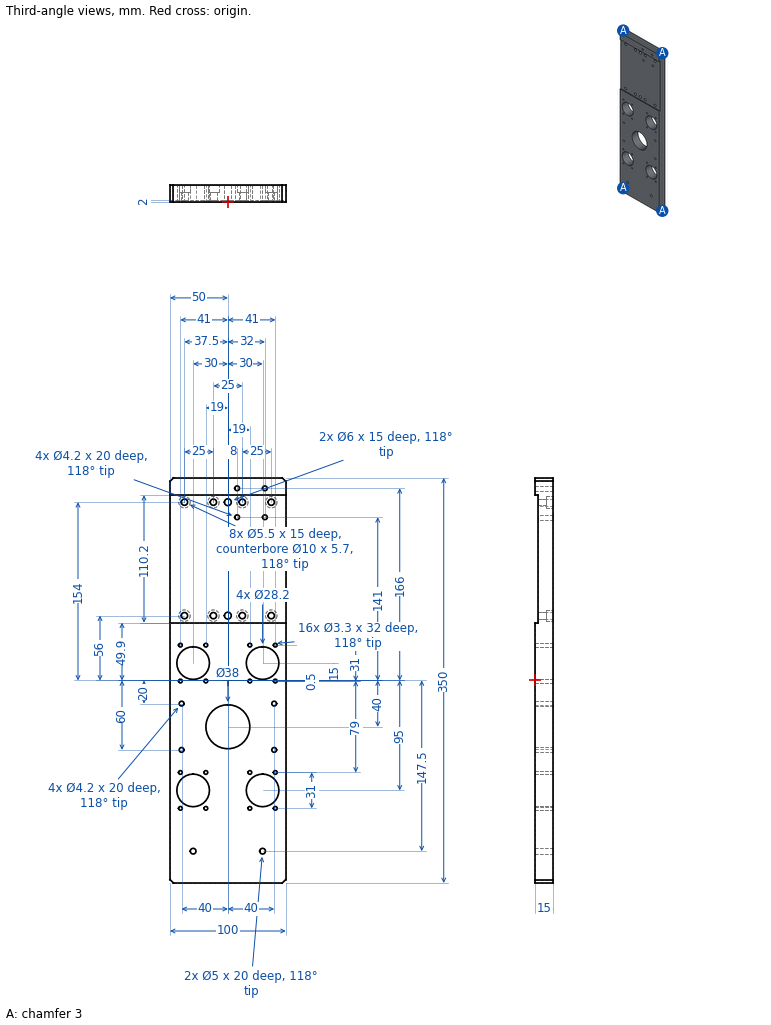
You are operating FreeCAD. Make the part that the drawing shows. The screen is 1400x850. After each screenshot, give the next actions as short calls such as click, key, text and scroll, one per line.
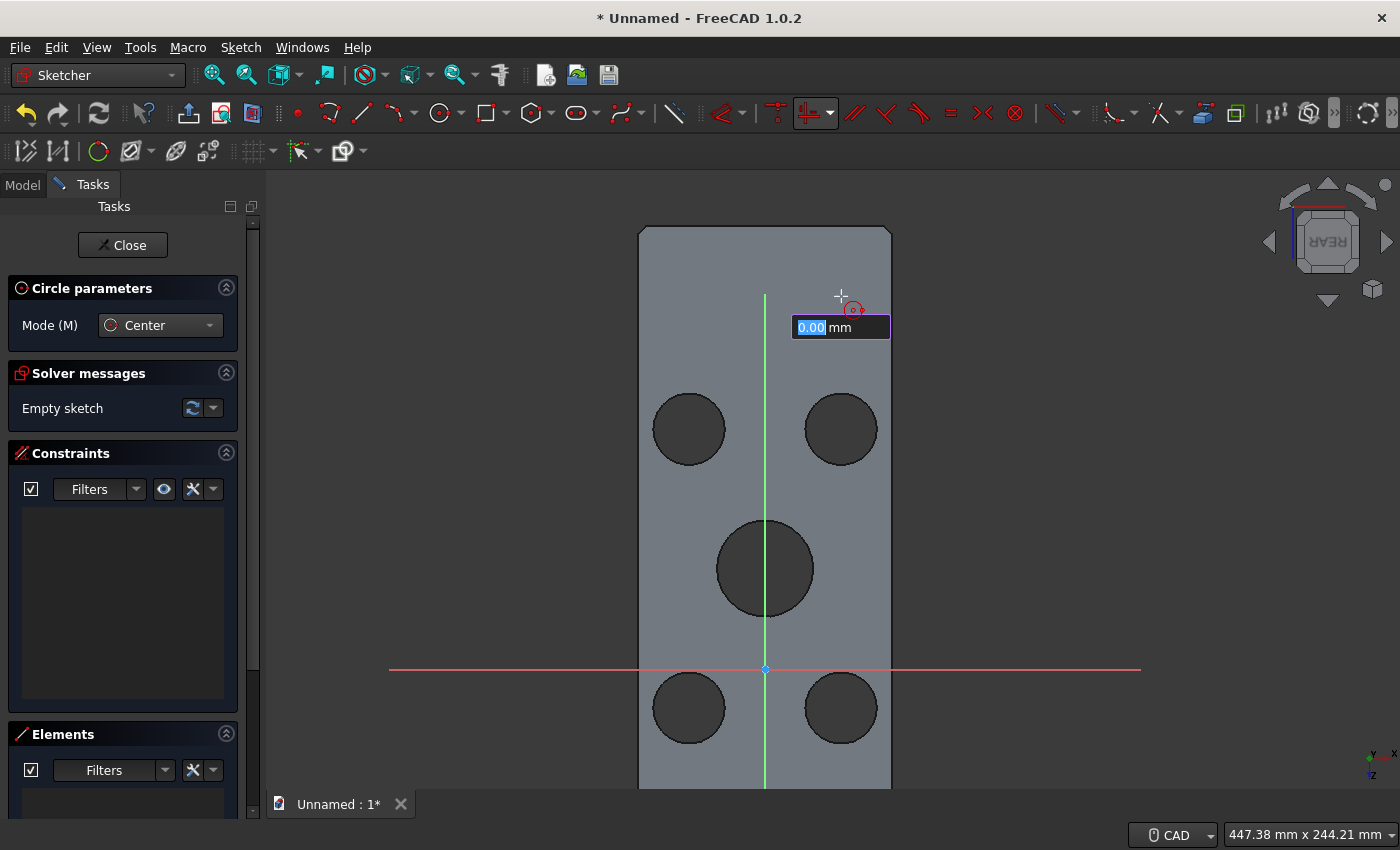
scroll(846, 292, up, 5)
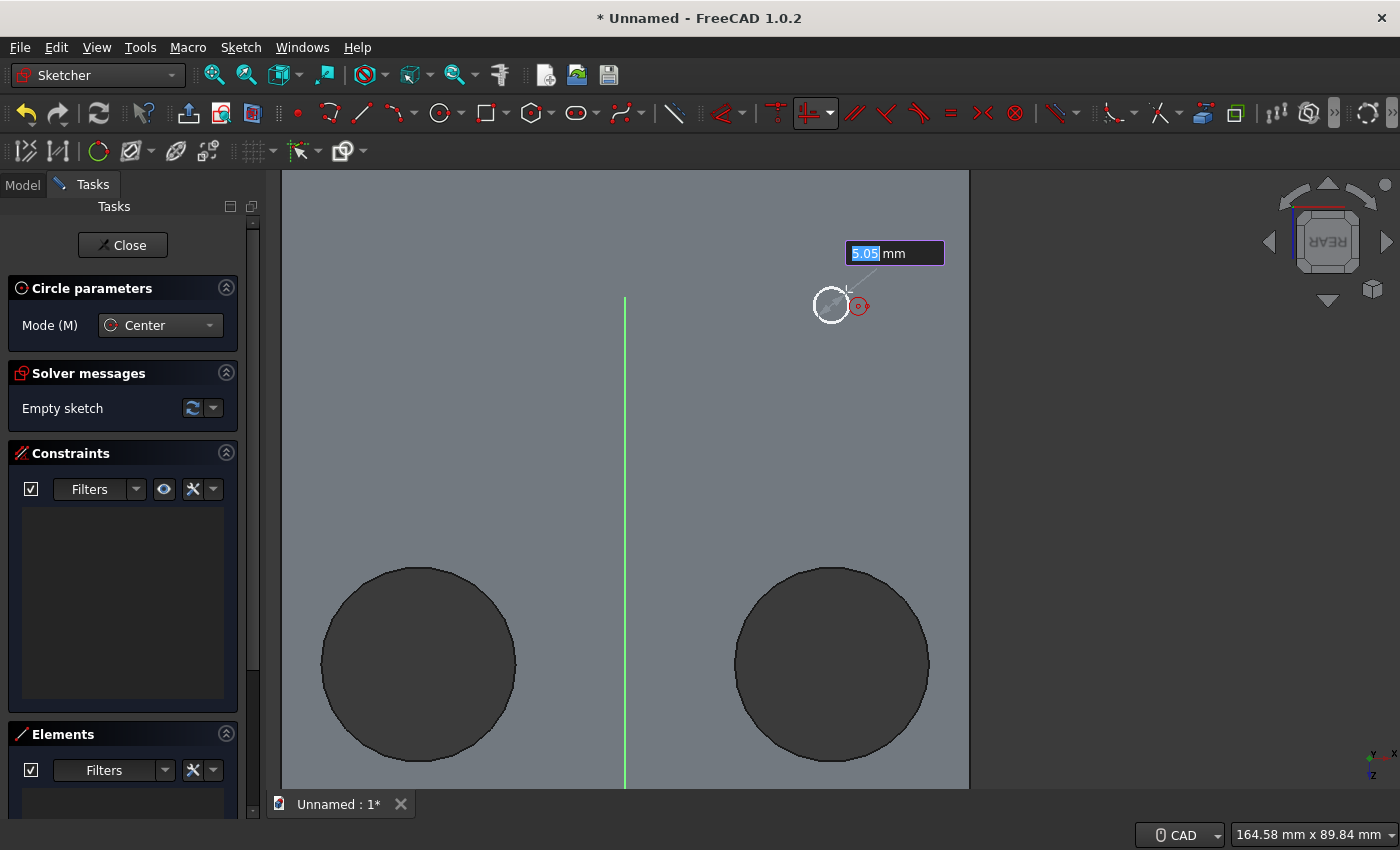
click(844, 291)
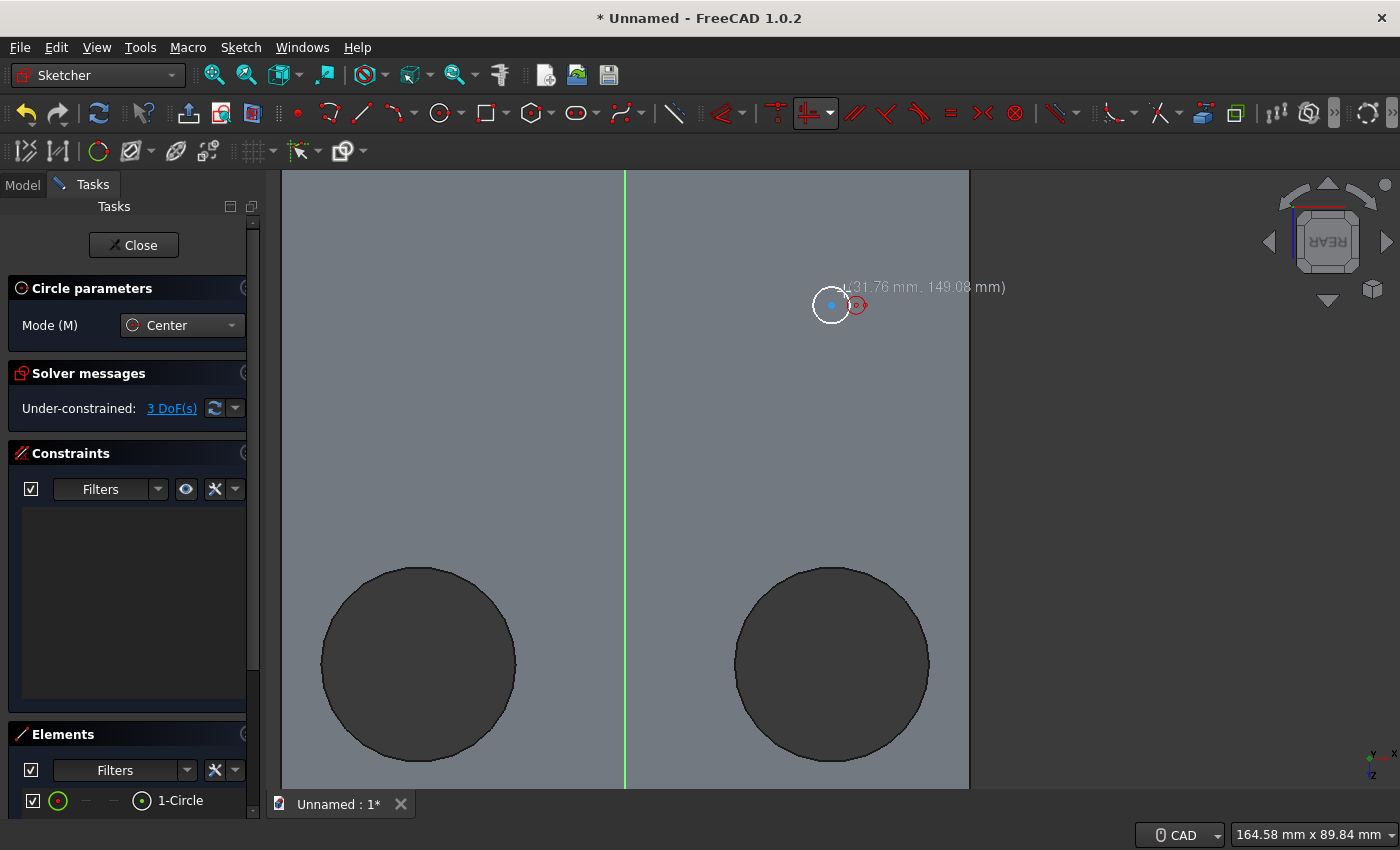
scroll(418, 303, up, 2)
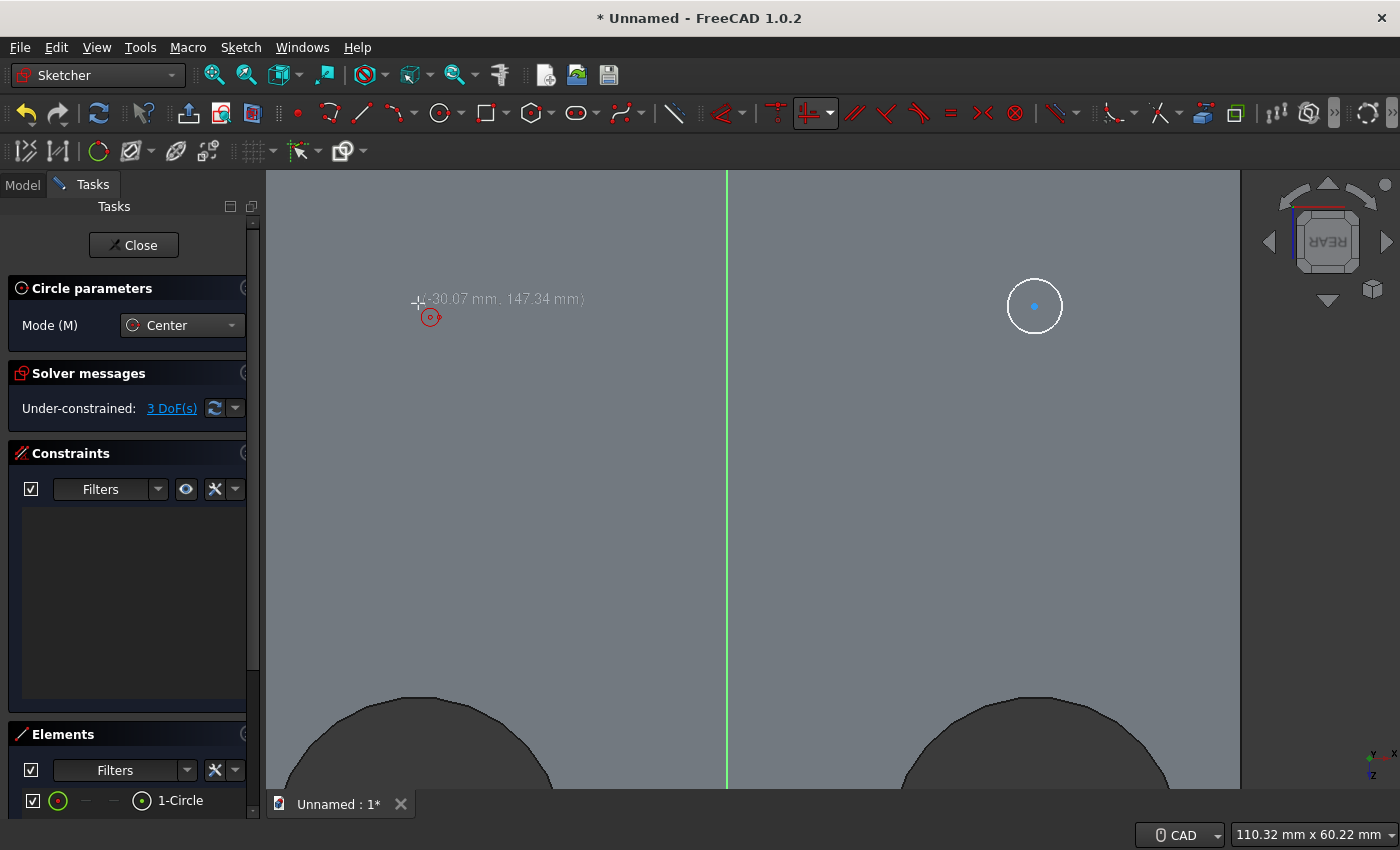
scroll(777, 293, down, 7)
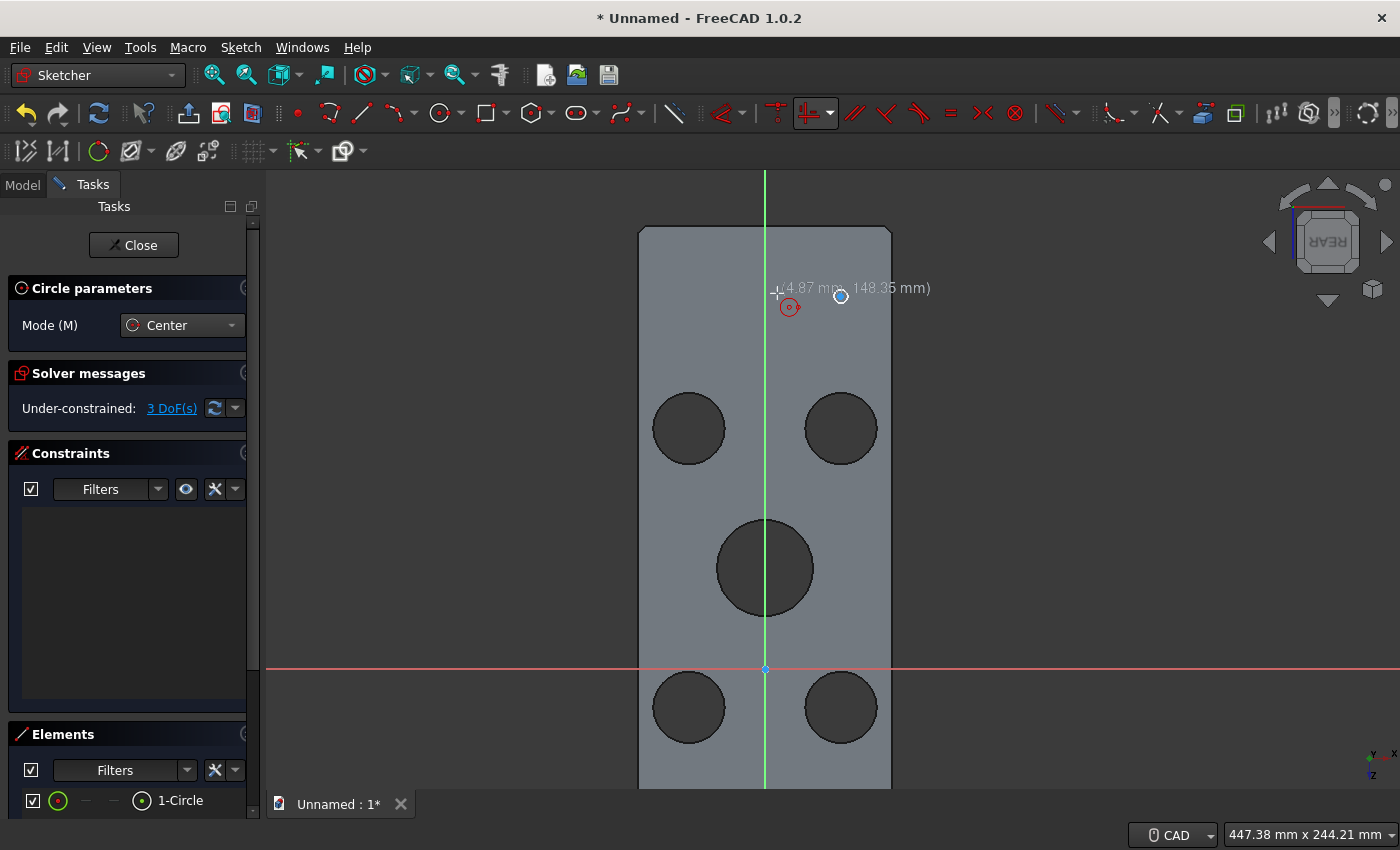
click(689, 296)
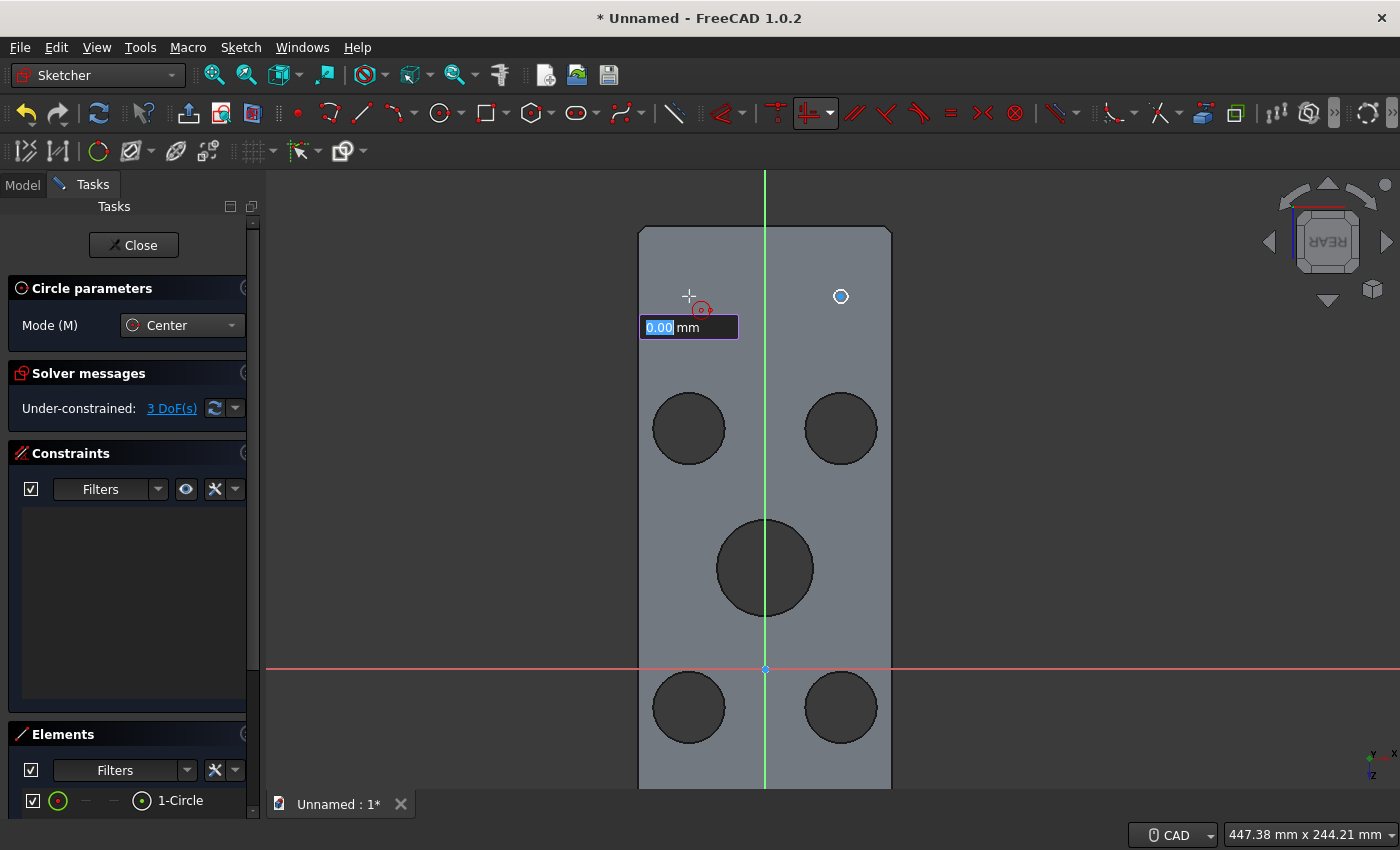
scroll(693, 291, up, 5)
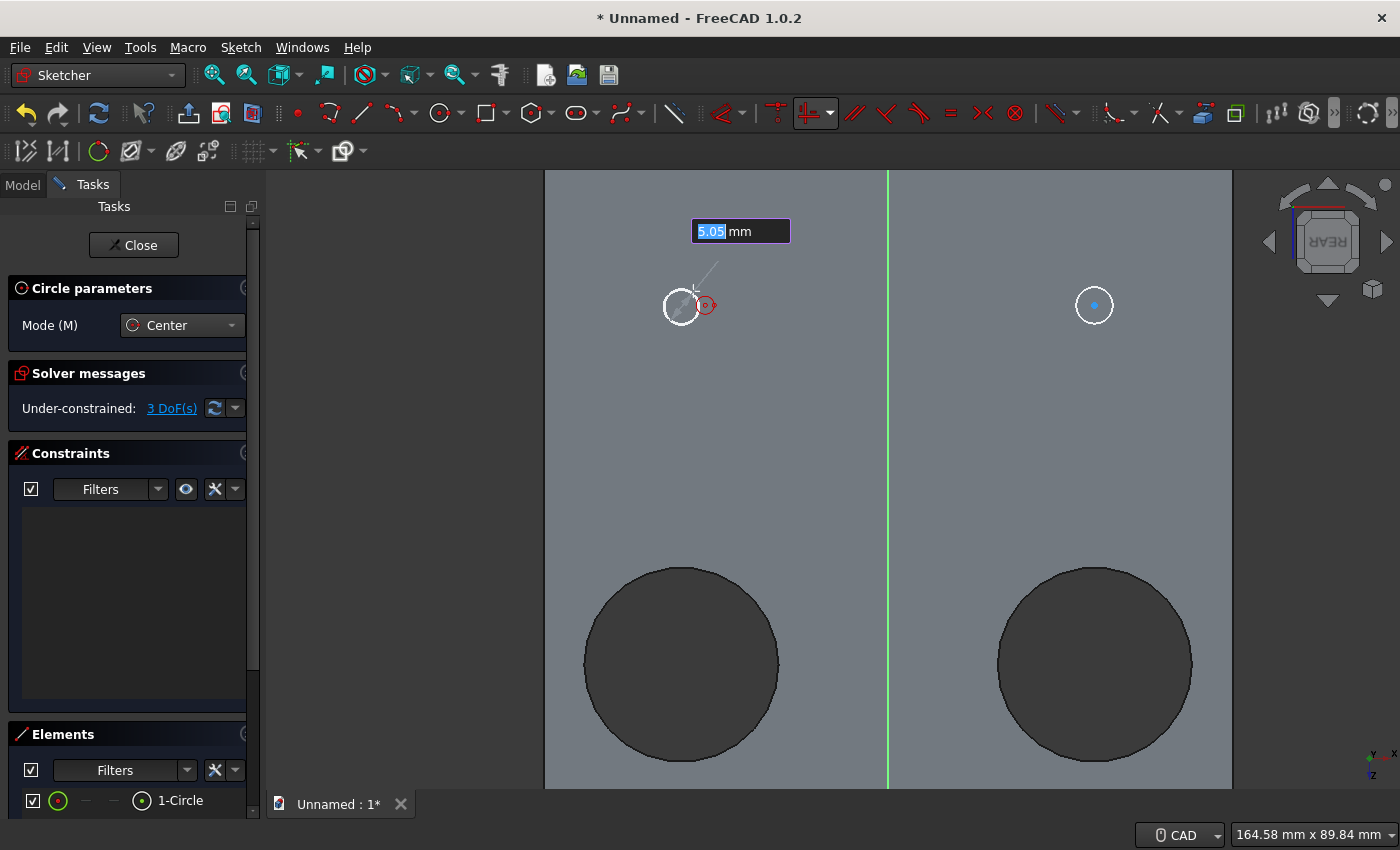
click(694, 291)
key(Escape)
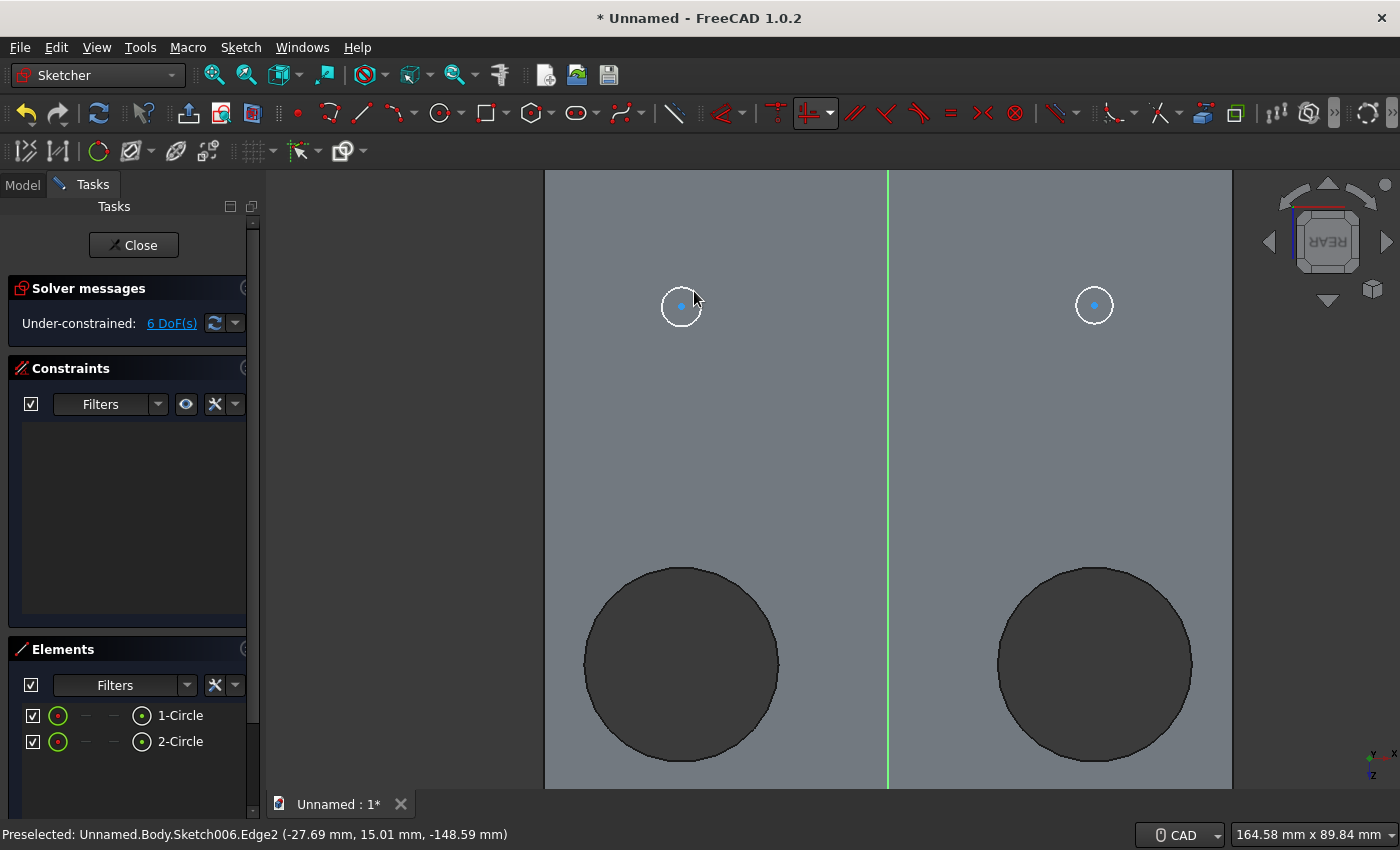
click(1107, 292)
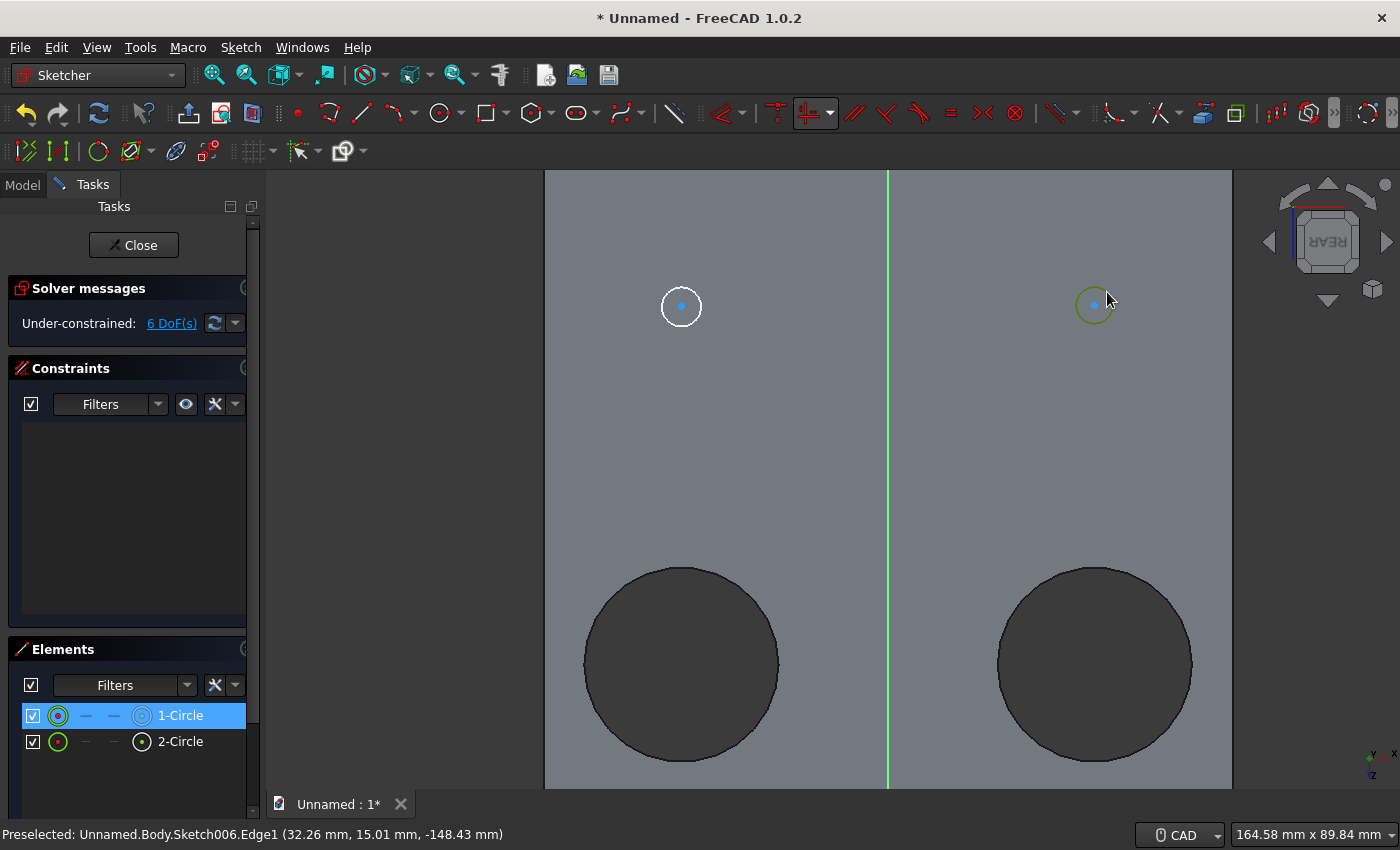
click(695, 293)